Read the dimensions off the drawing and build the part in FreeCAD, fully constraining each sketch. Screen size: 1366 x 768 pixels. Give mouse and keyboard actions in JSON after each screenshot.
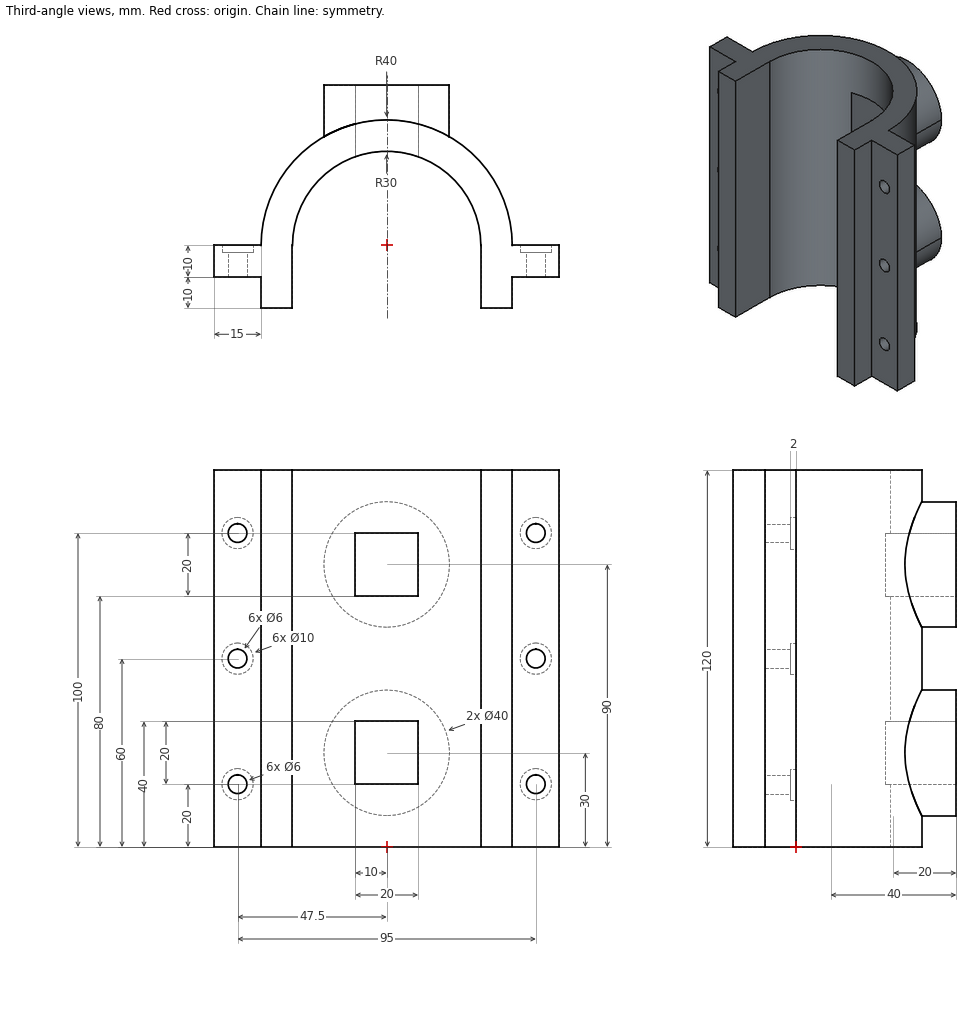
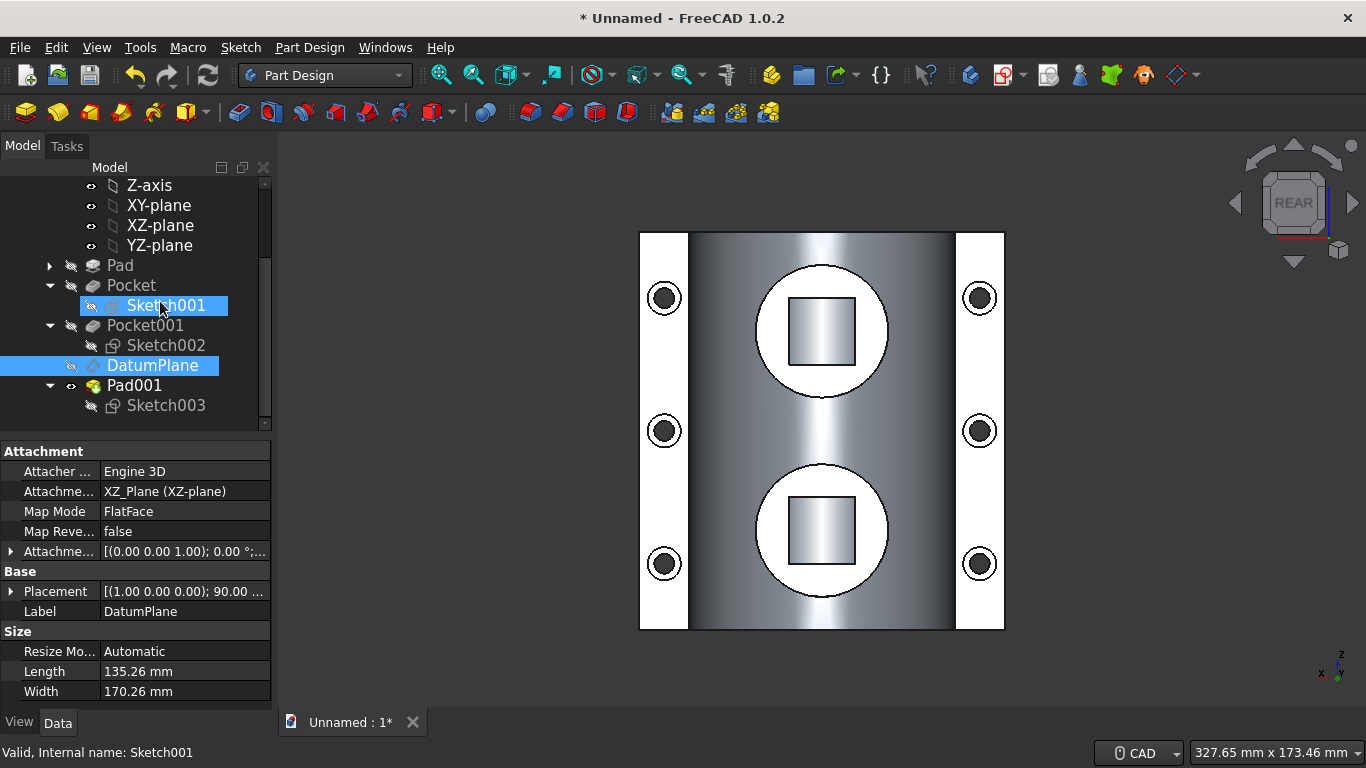
{"action": "scroll", "coordinate": [160, 301], "scroll_direction": "up", "scroll_amount": 15}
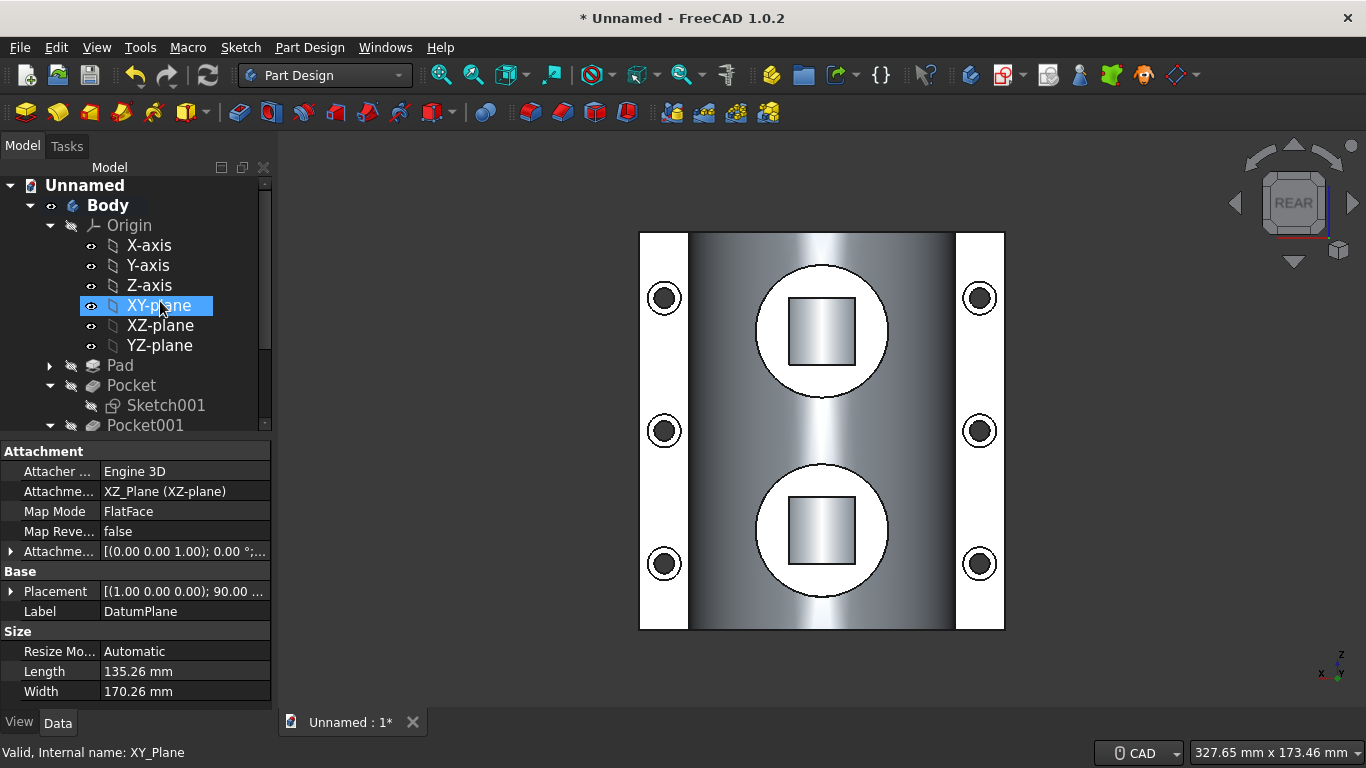
{"action": "left_click", "coordinate": [136, 326]}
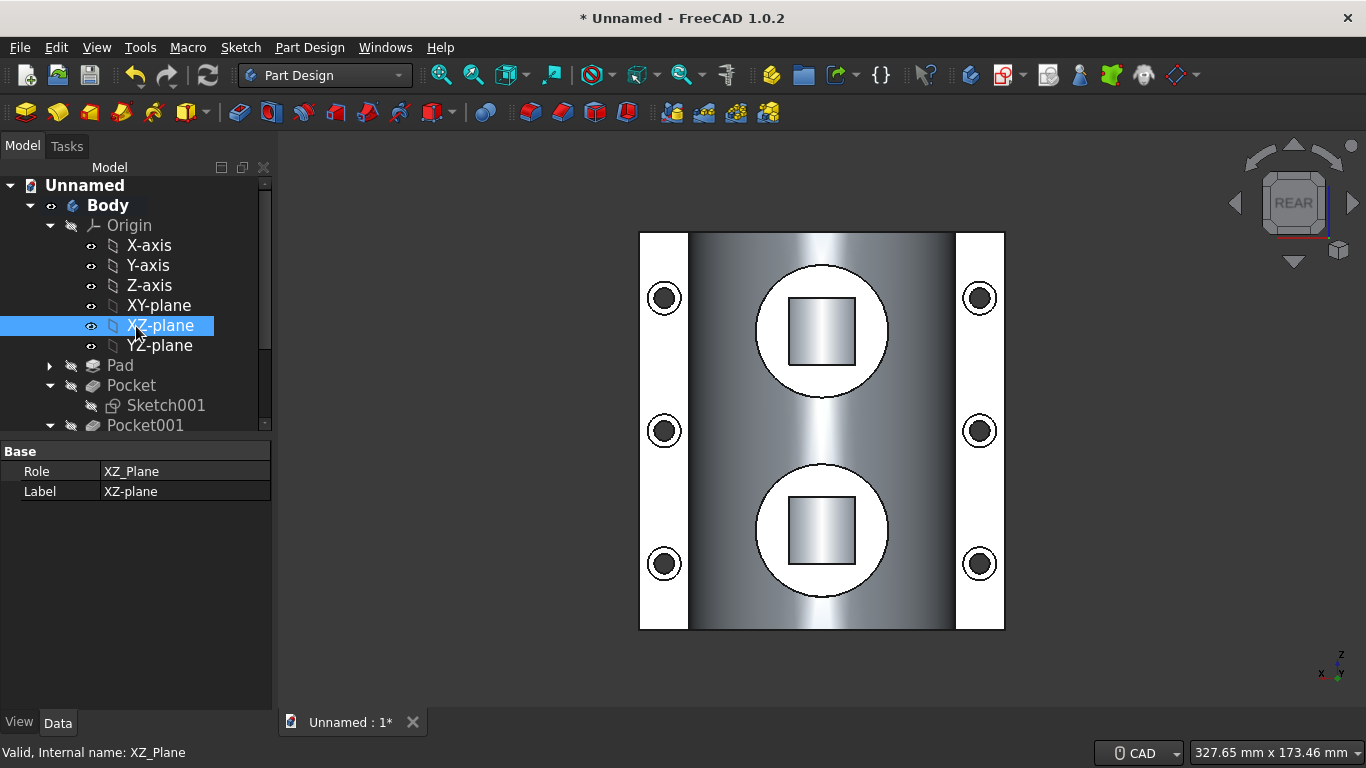
{"action": "left_click", "coordinate": [1176, 76]}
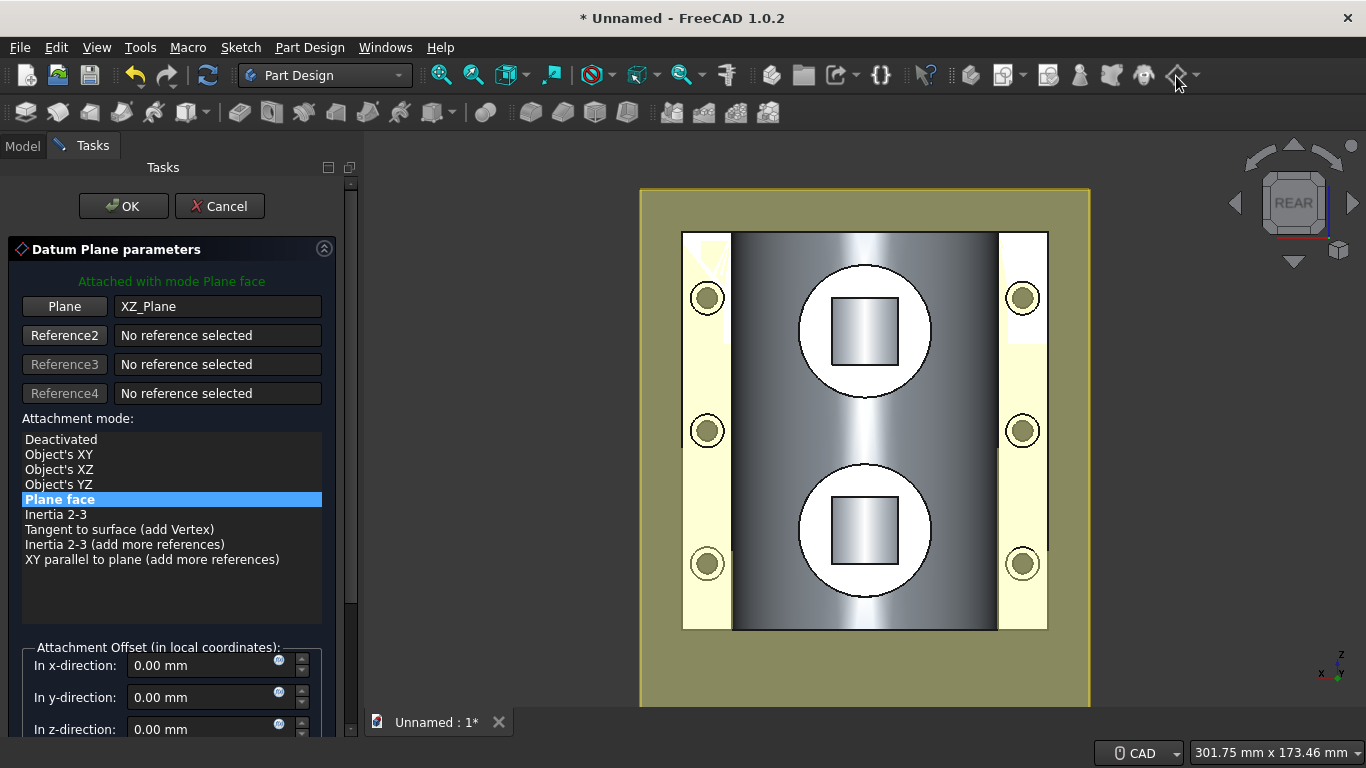
{"action": "scroll", "coordinate": [351, 456], "scroll_direction": "down", "scroll_amount": 2}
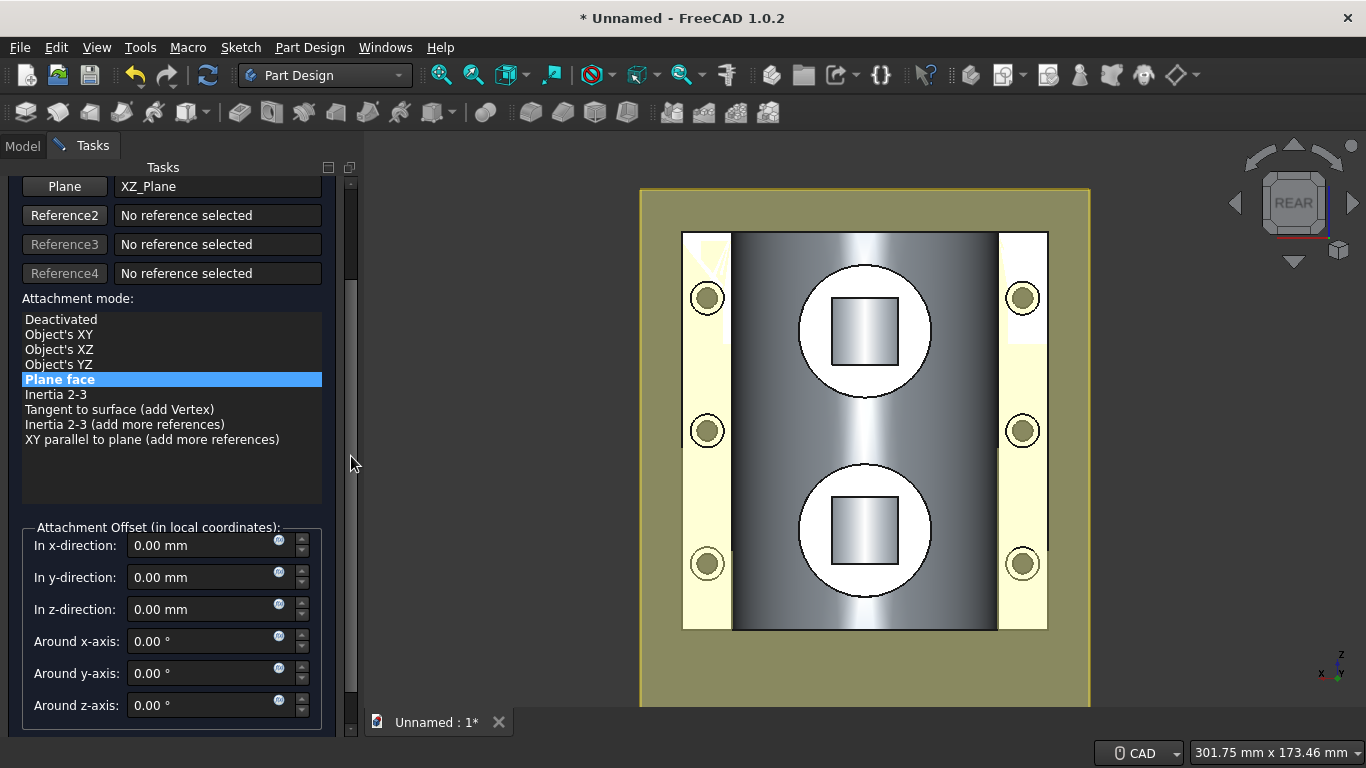
{"action": "triple_click", "coordinate": [210, 609]}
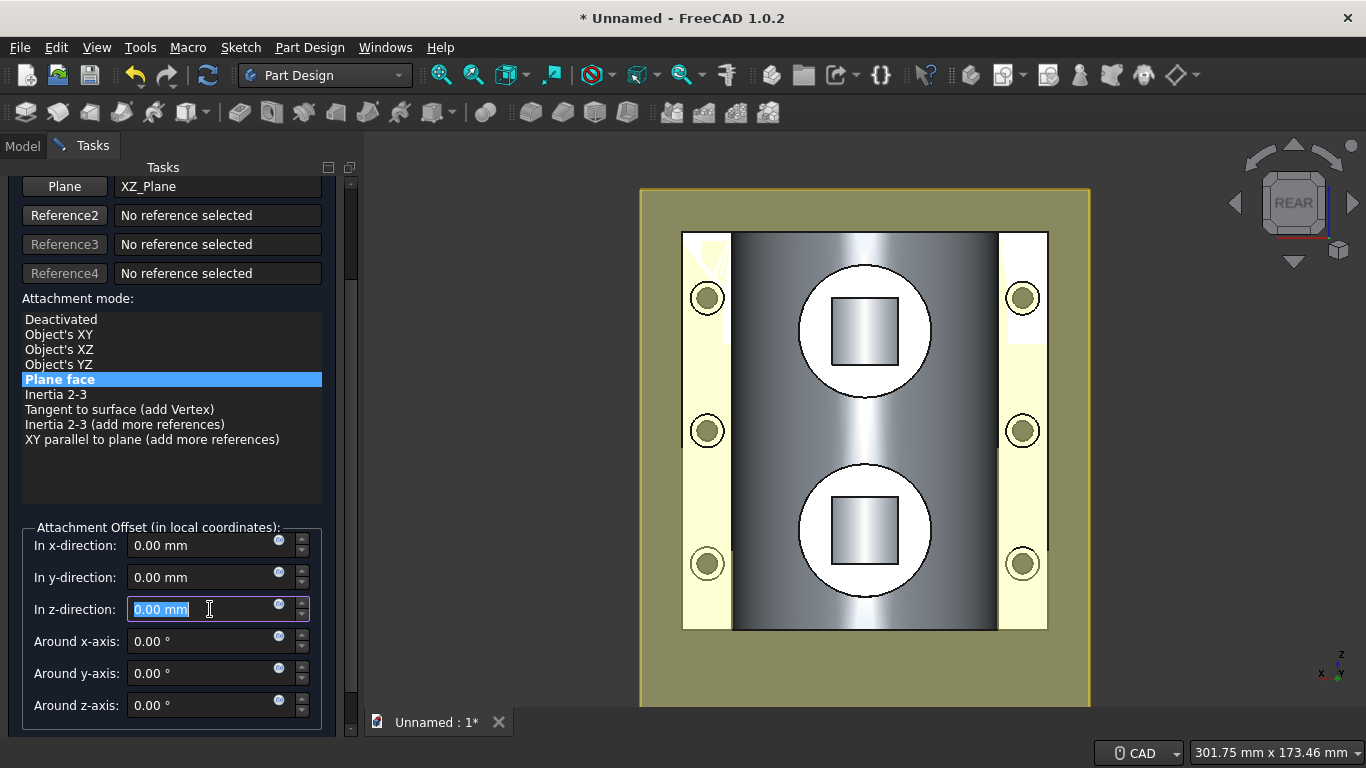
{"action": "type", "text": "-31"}
{"action": "key", "text": "Tab"}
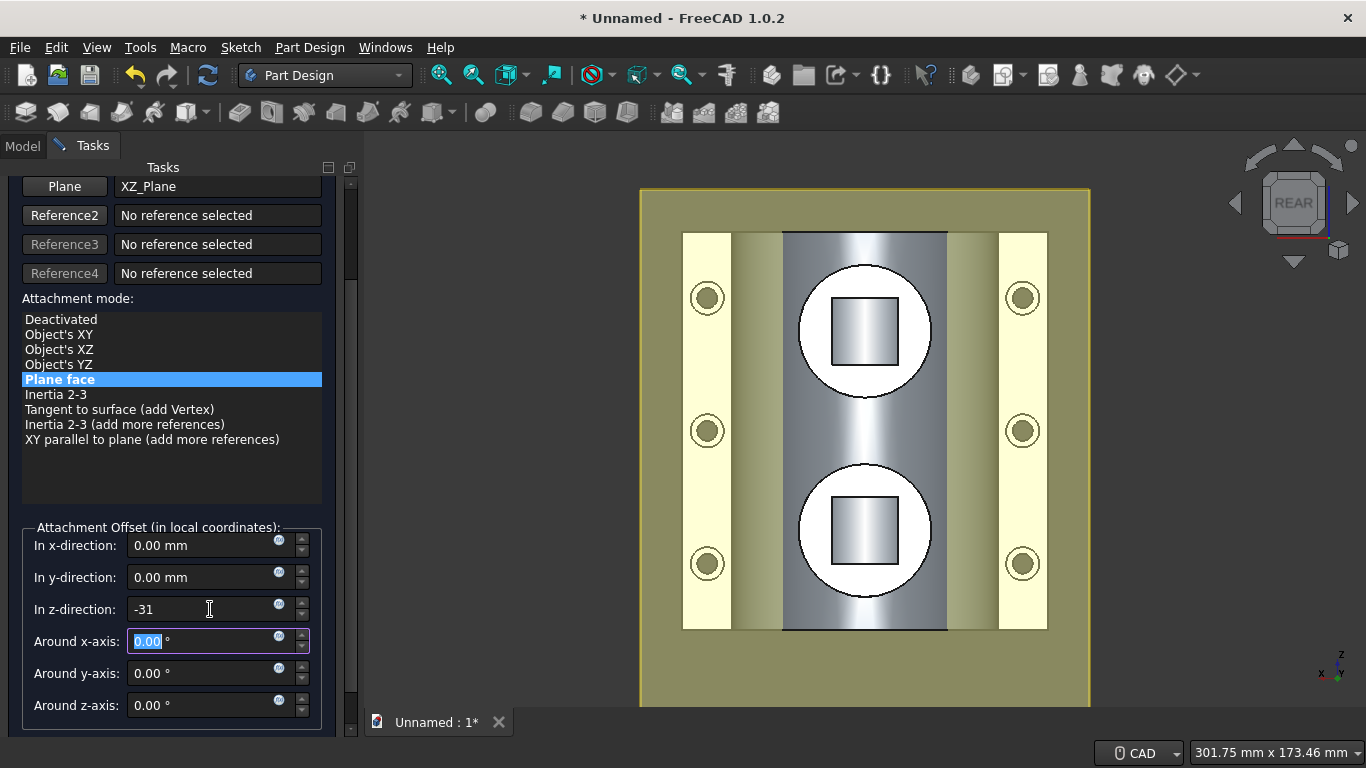
{"action": "scroll", "coordinate": [351, 456], "scroll_direction": "up", "scroll_amount": 3}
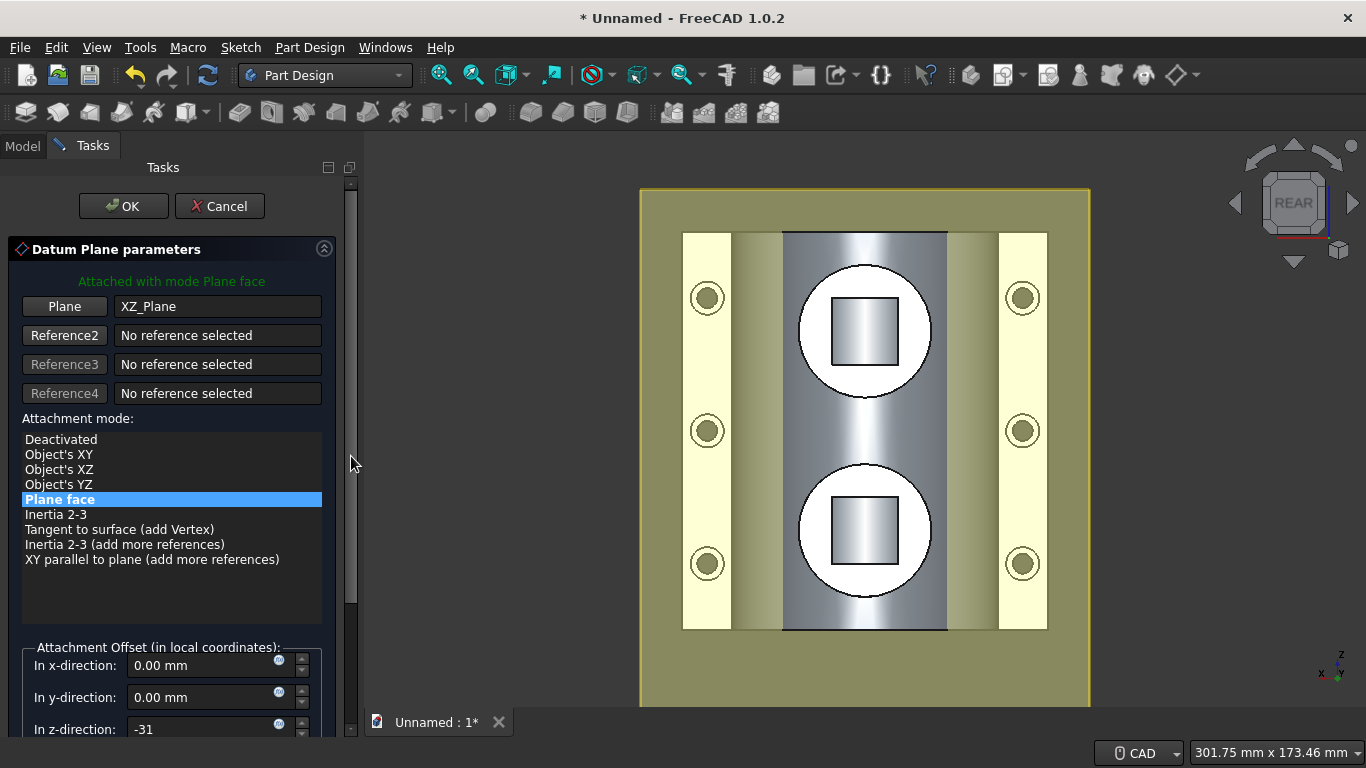
{"action": "left_click", "coordinate": [124, 206]}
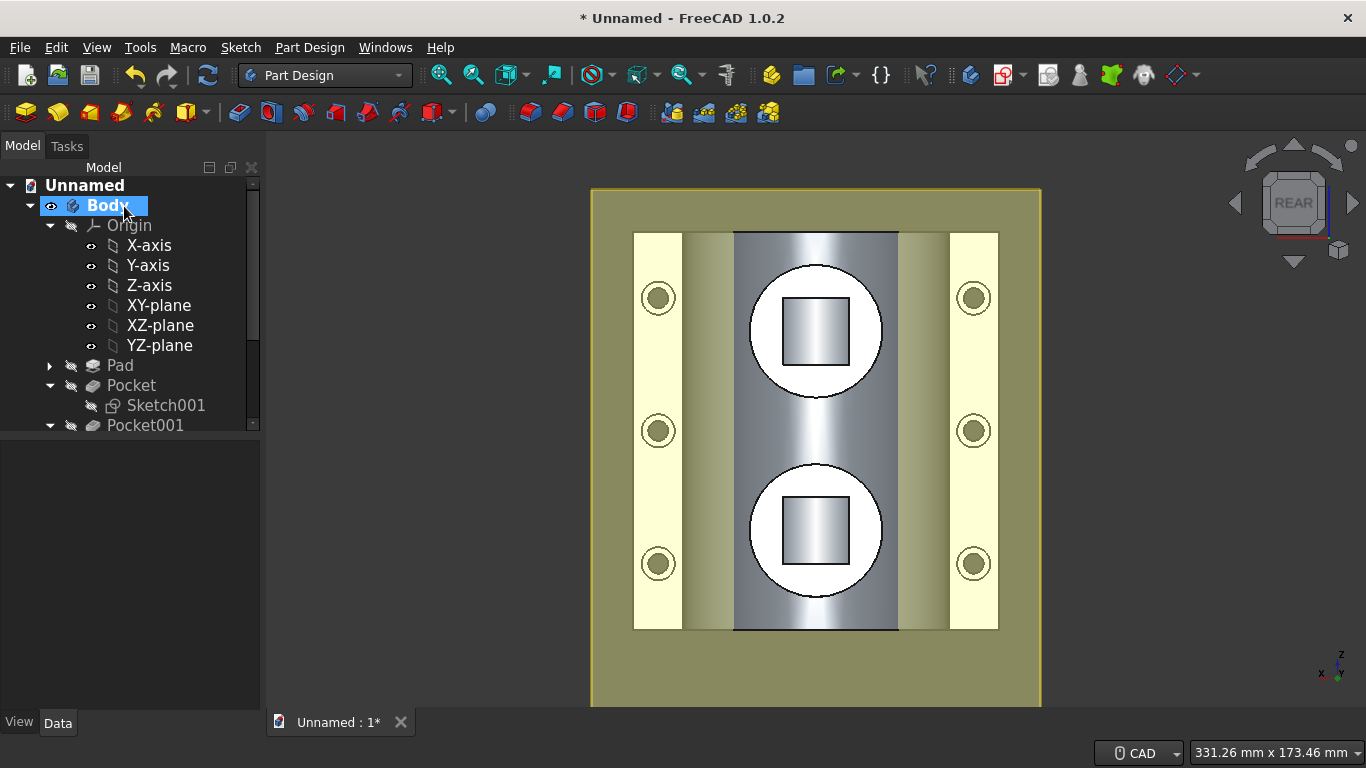
{"action": "scroll", "coordinate": [100, 301], "scroll_direction": "down", "scroll_amount": 3}